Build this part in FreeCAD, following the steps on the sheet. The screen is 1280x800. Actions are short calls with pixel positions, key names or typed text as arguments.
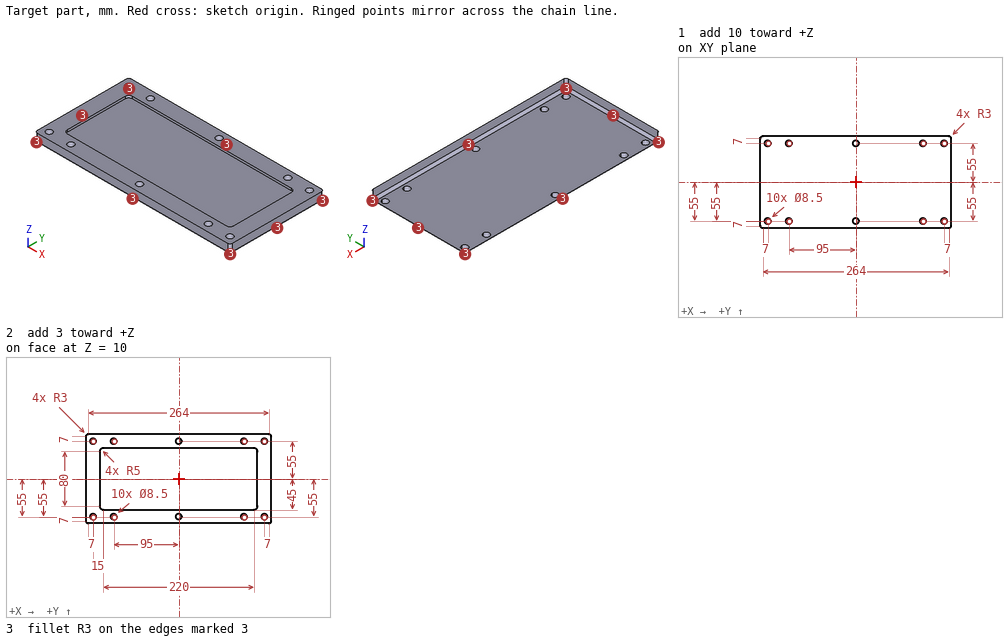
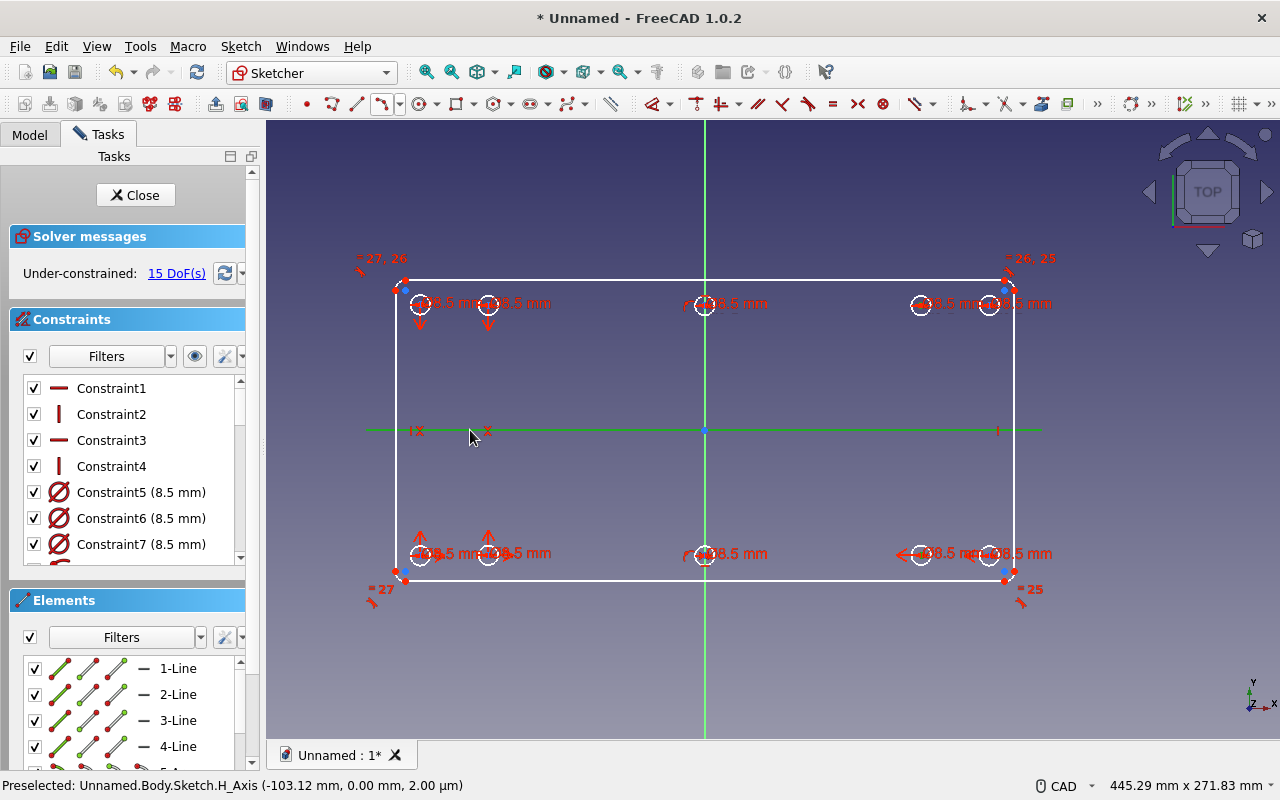
click(858, 104)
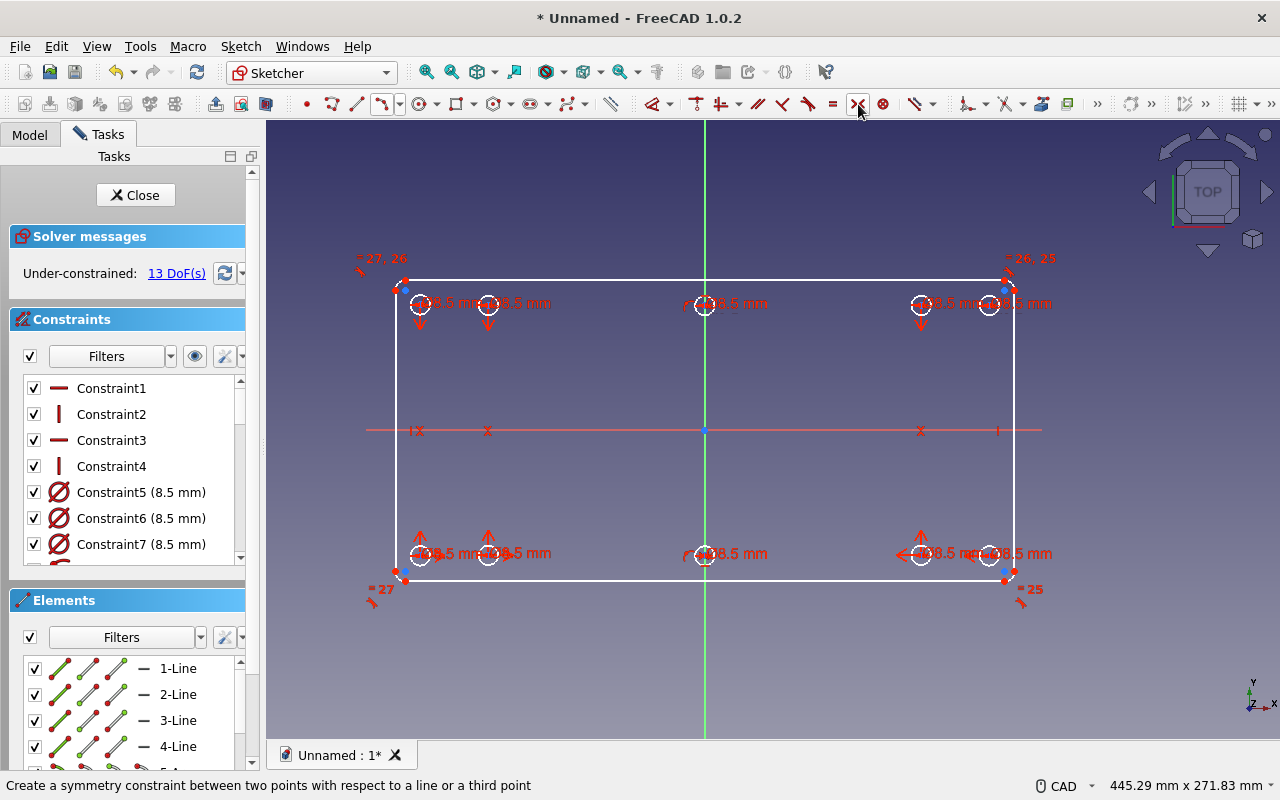
click(989, 556)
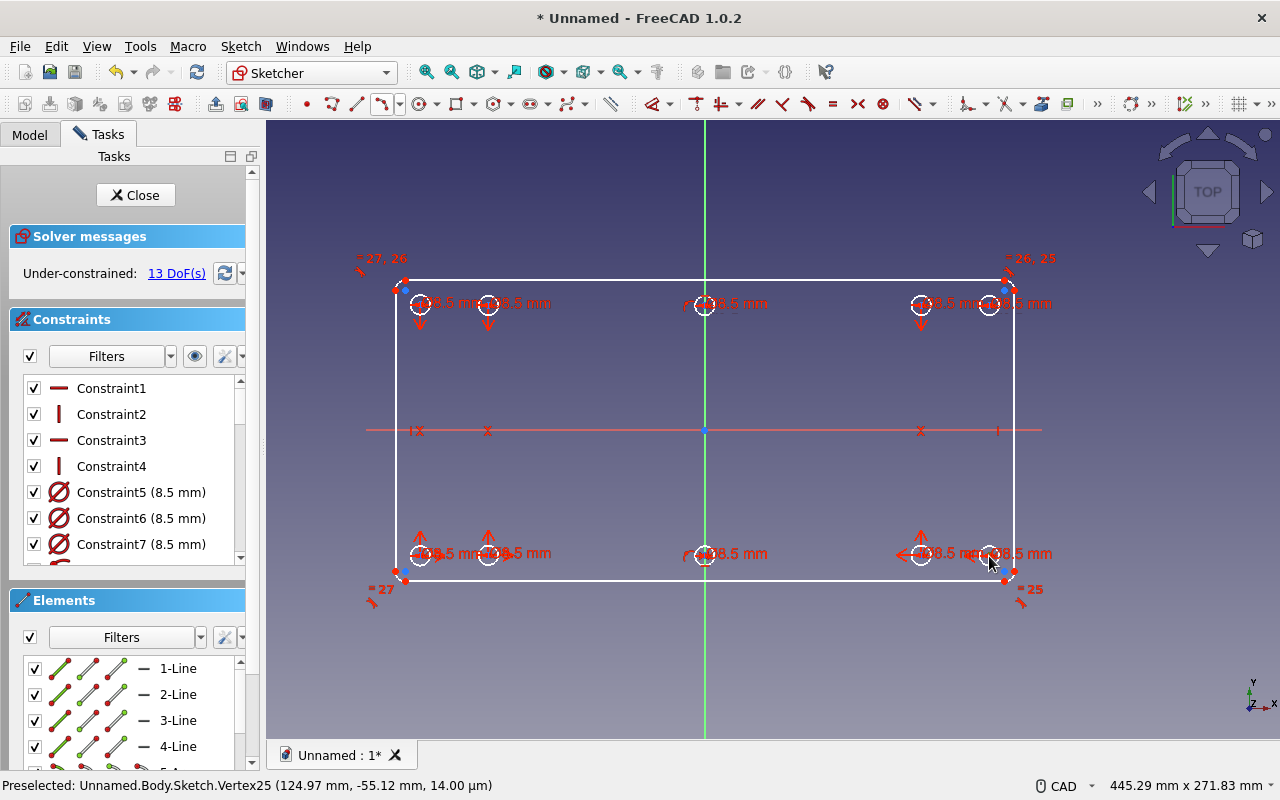
click(989, 306)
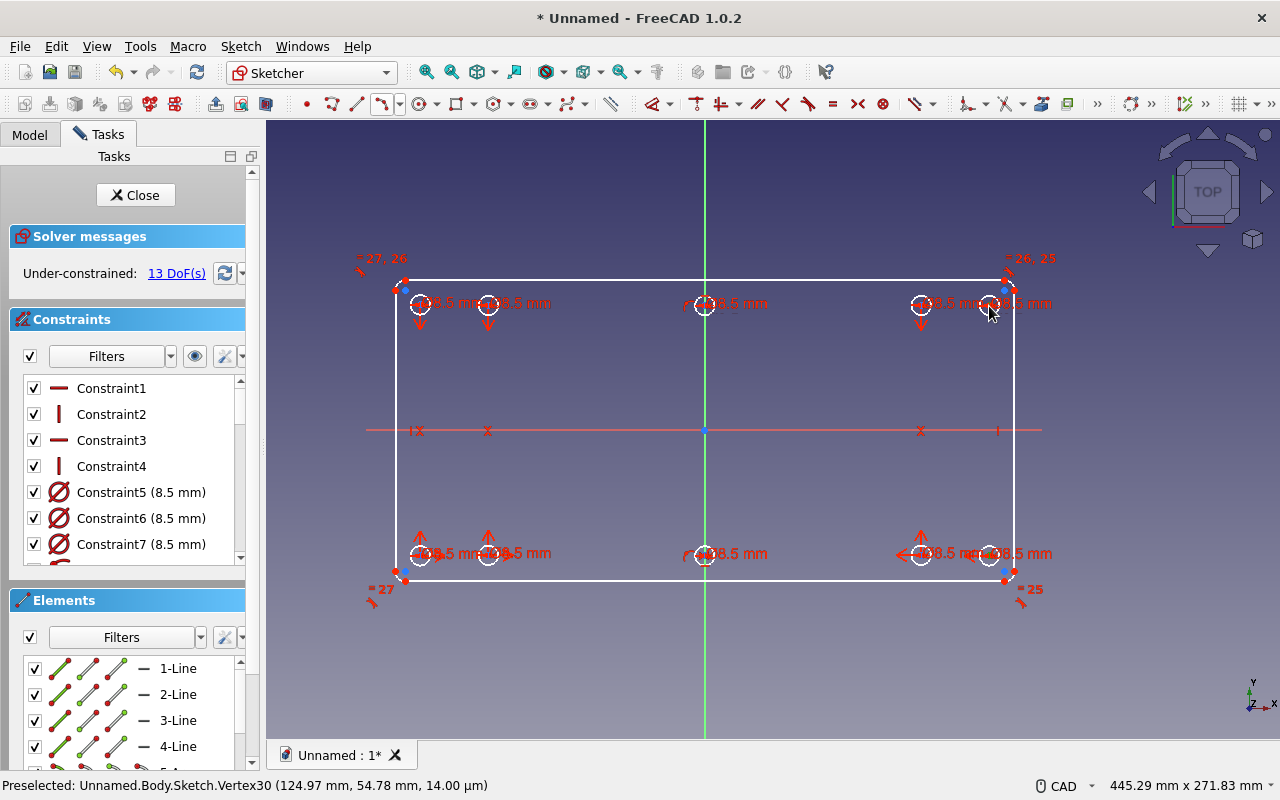
click(470, 430)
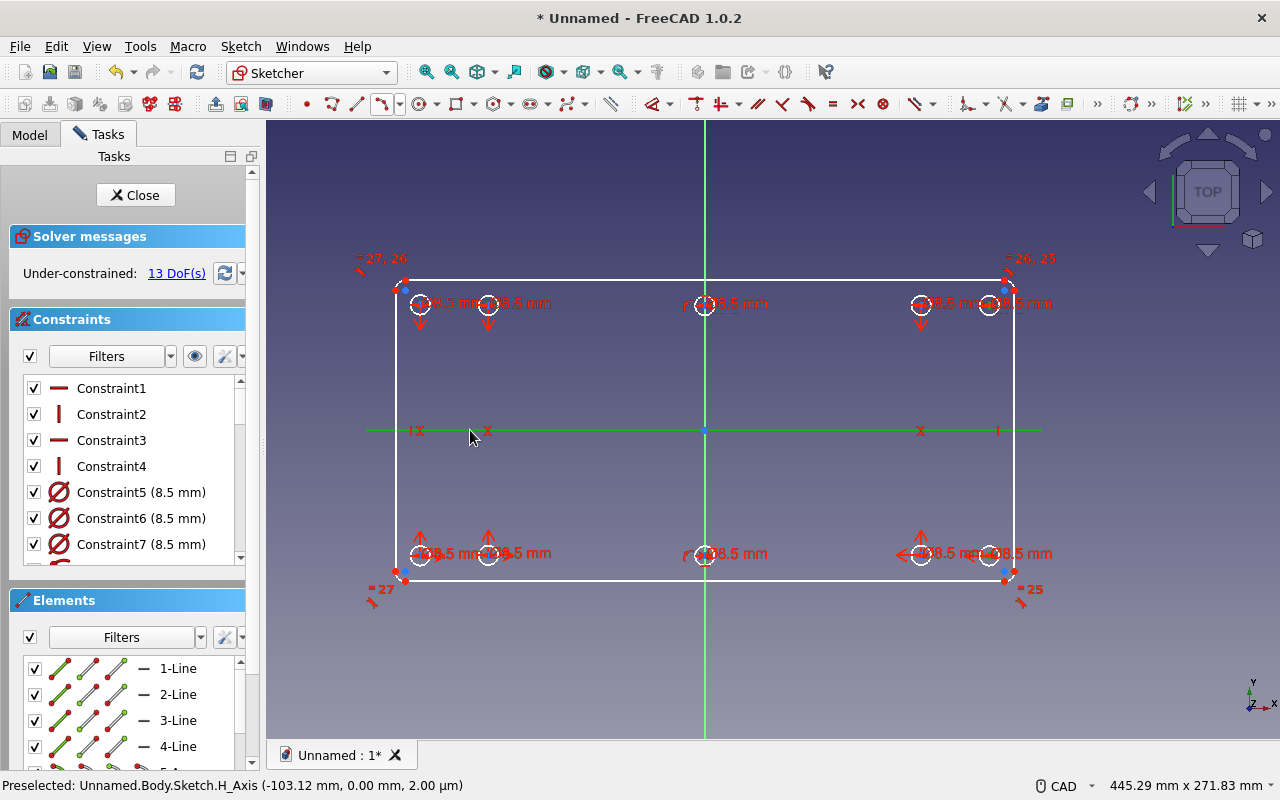
click(858, 104)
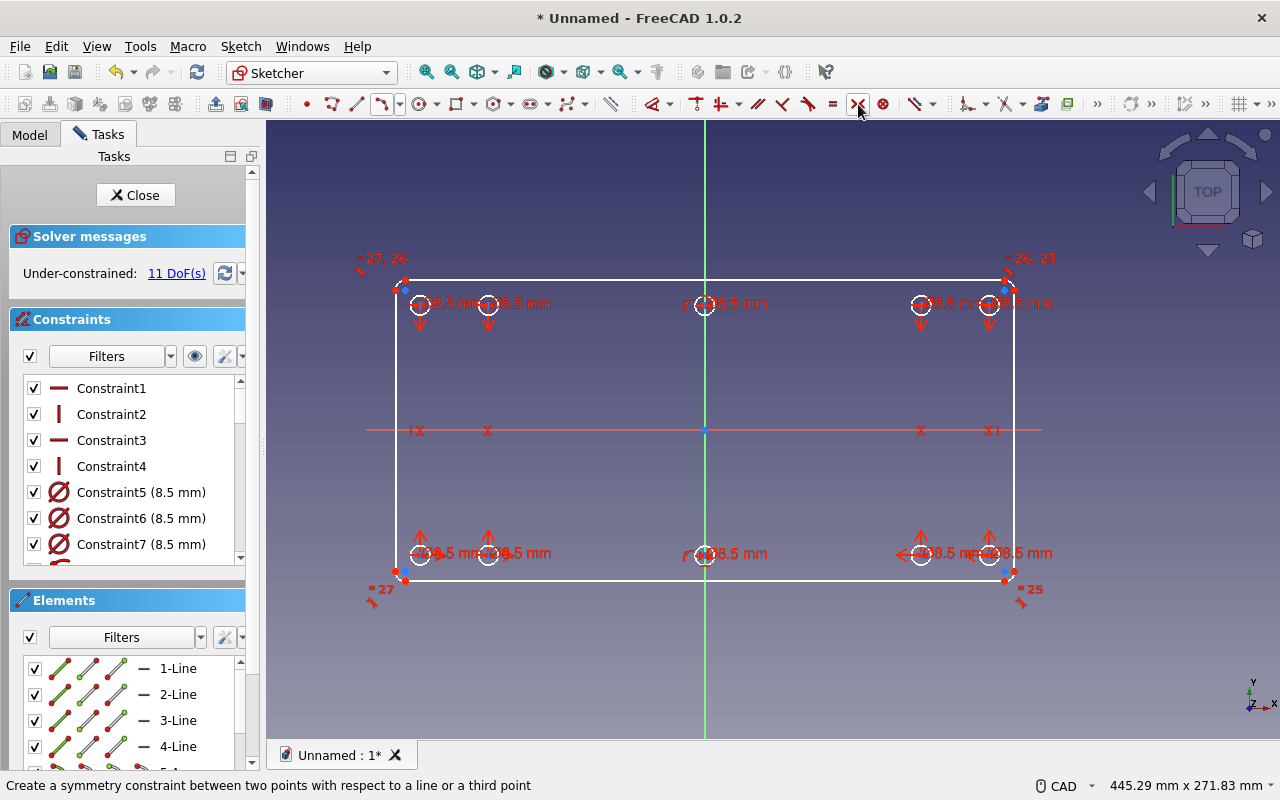
click(652, 104)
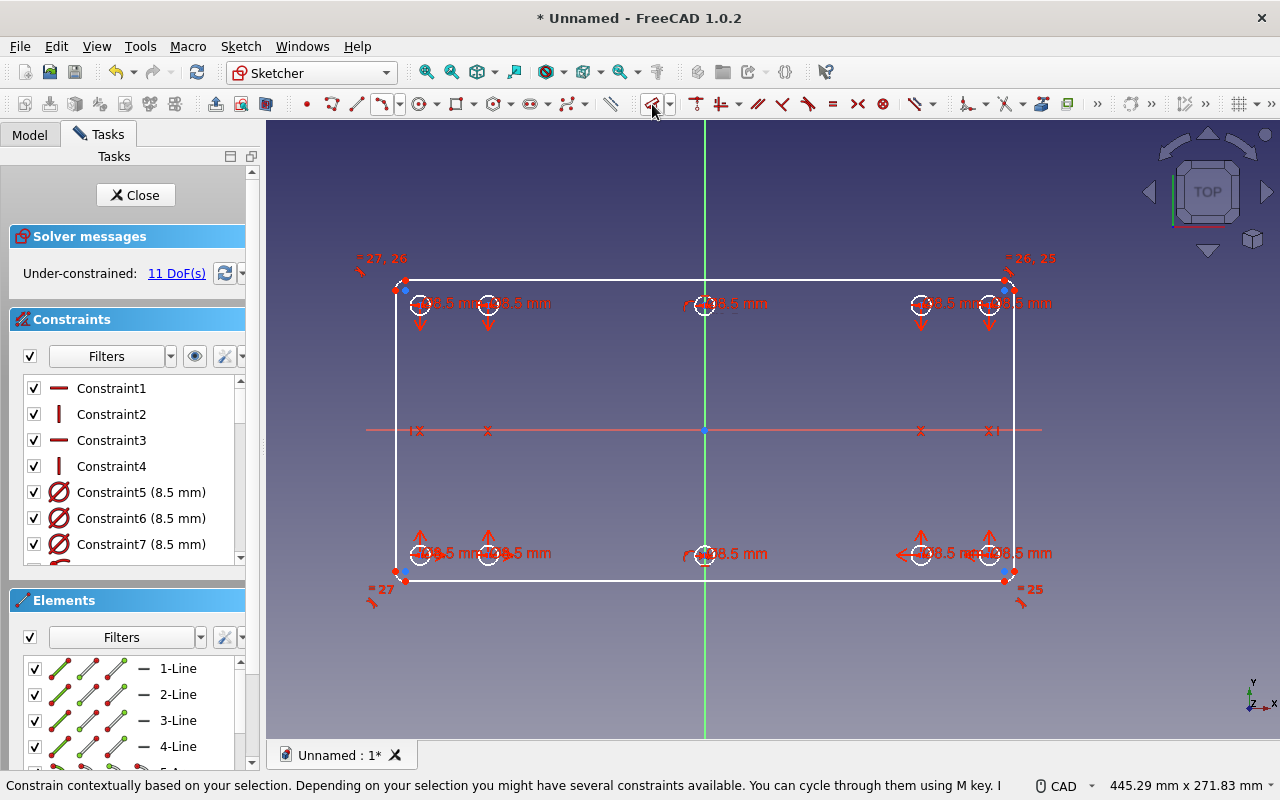
scroll(1012, 579, up, 9)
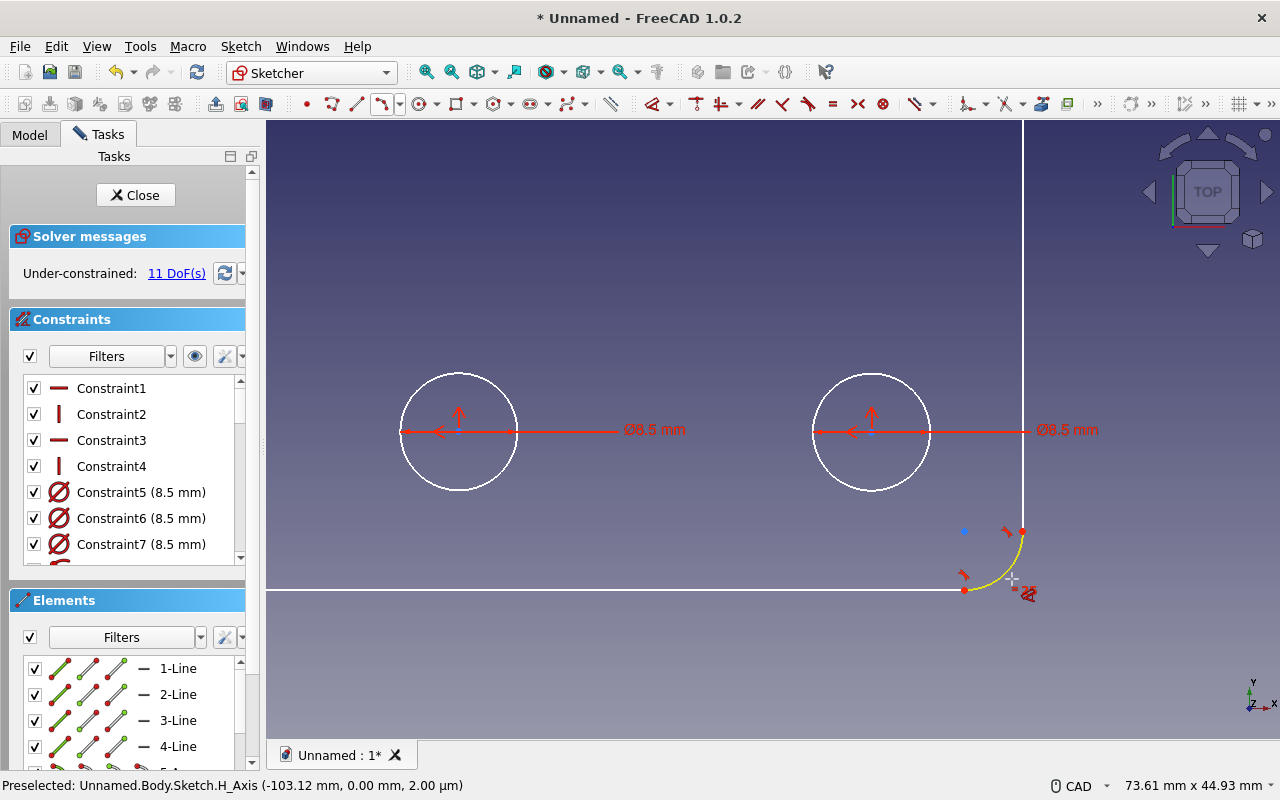
click(1006, 573)
click(1029, 596)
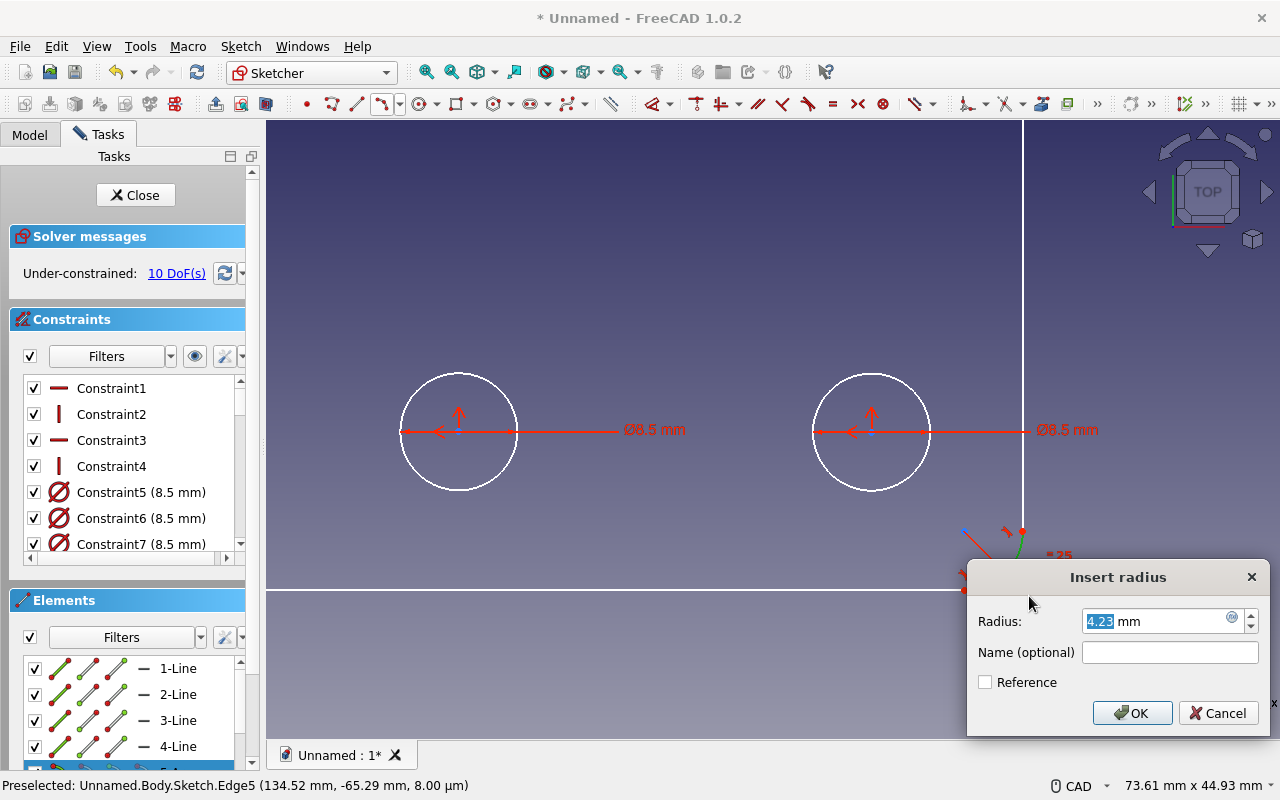
text(3)
key(Return)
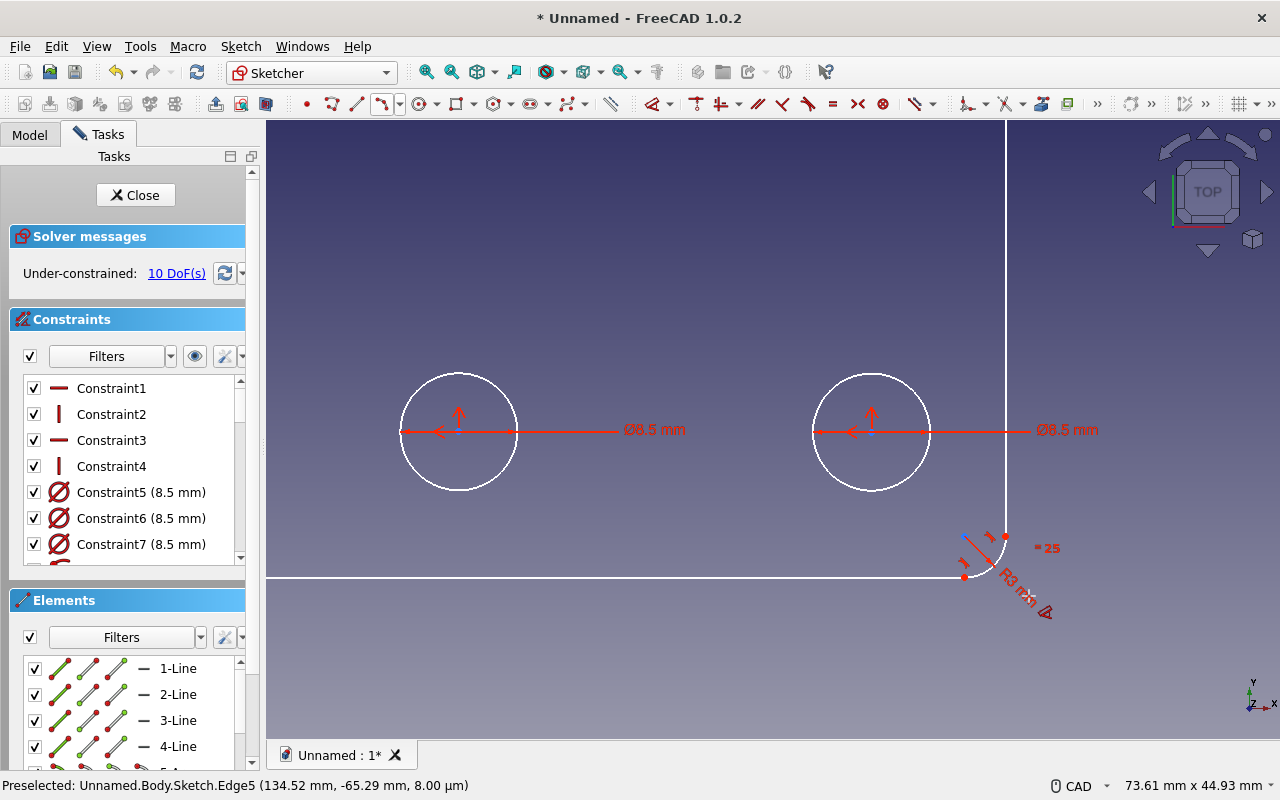
scroll(1012, 579, down, 9)